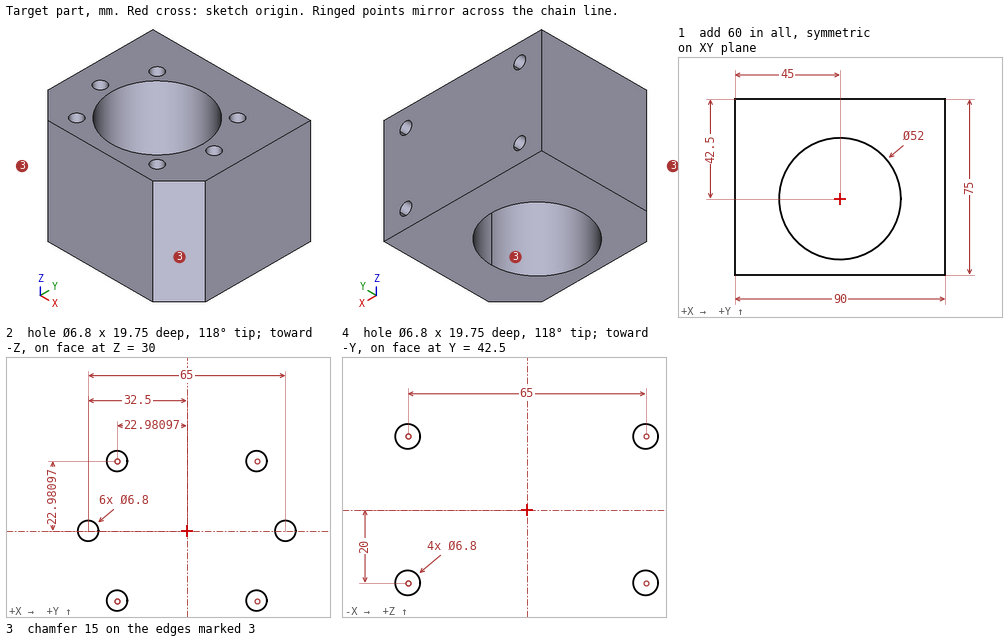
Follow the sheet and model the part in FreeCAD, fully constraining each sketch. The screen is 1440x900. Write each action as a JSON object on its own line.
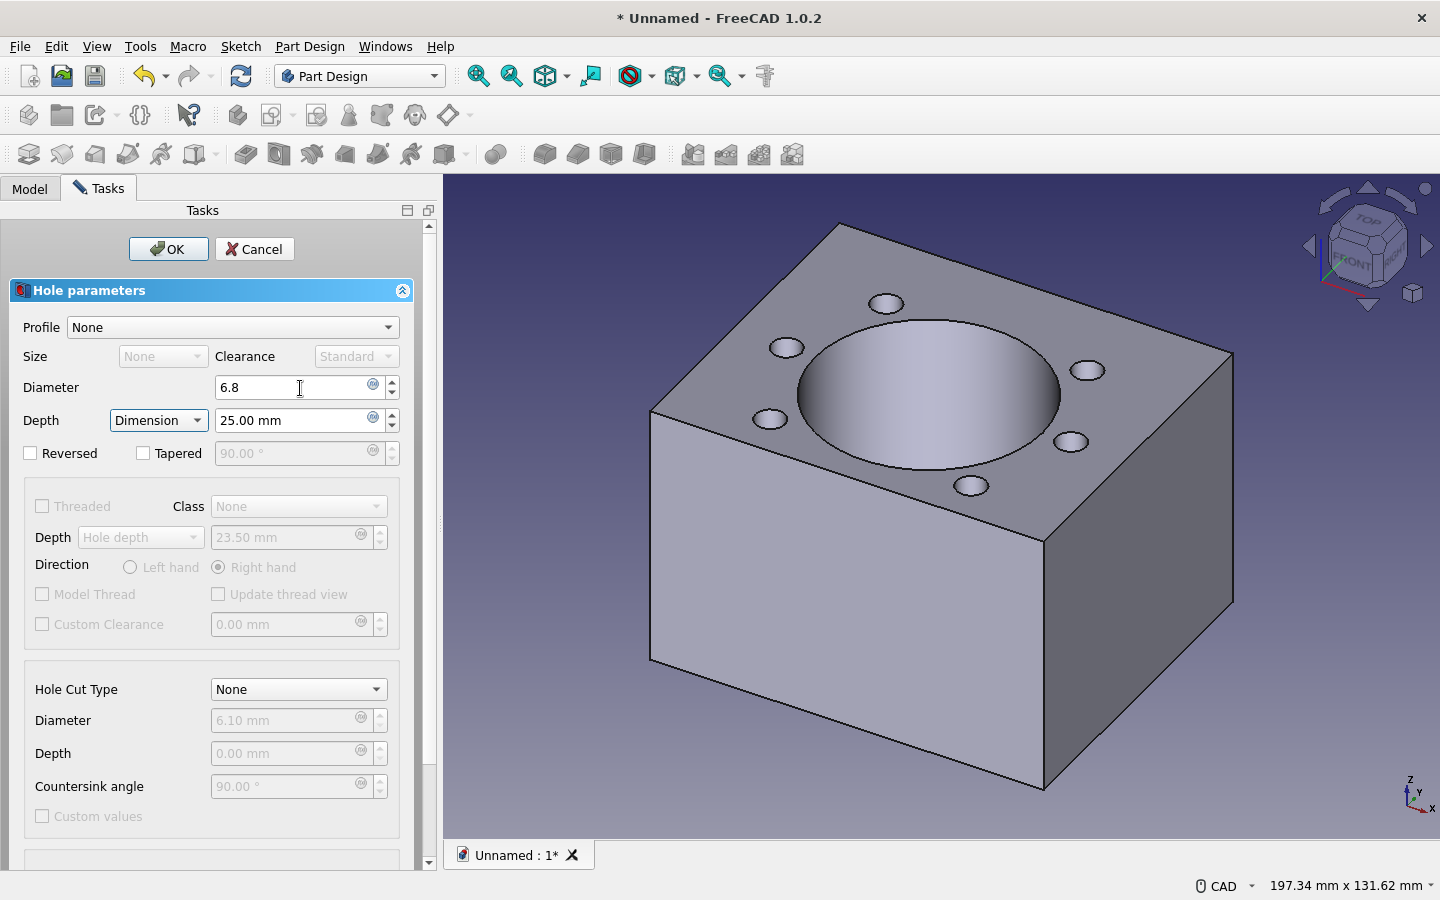
{"action": "triple_click", "coordinate": [300, 420]}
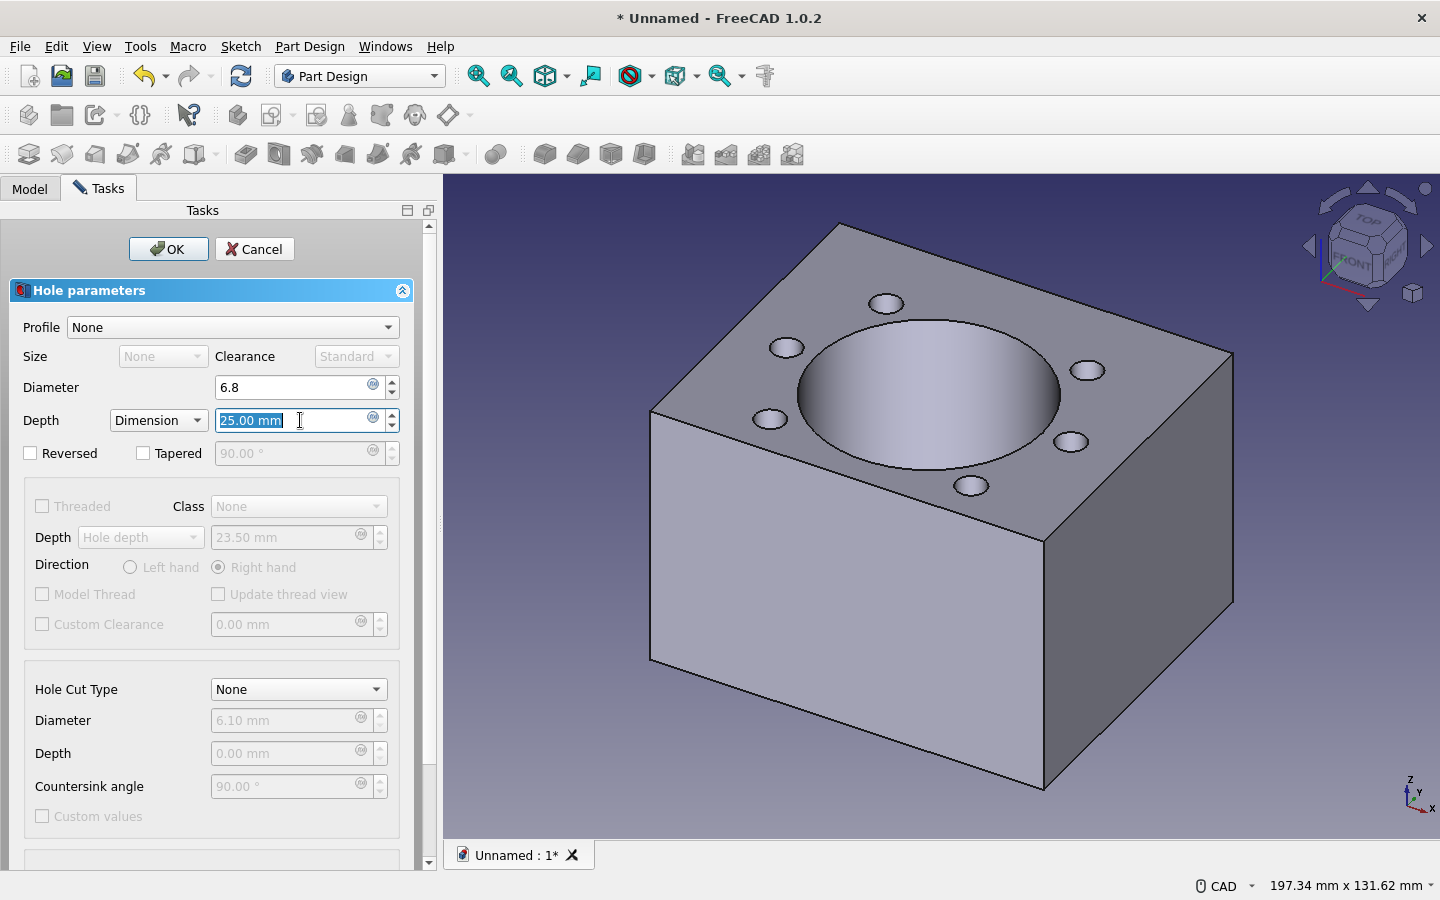
{"action": "type", "text": "19.75"}
{"action": "key", "text": "Tab"}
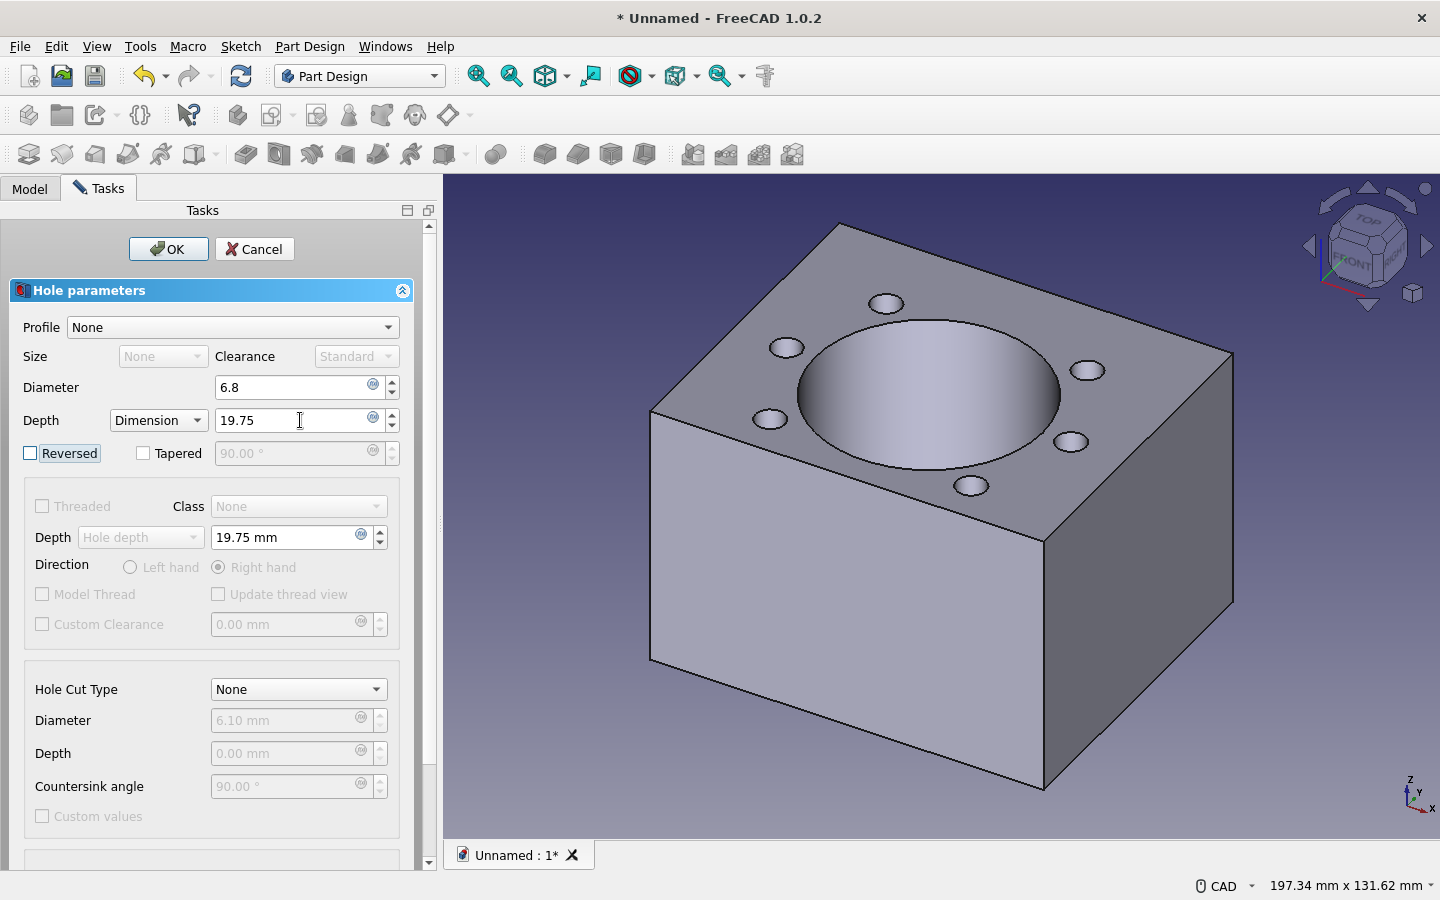
{"action": "left_click", "coordinate": [169, 249]}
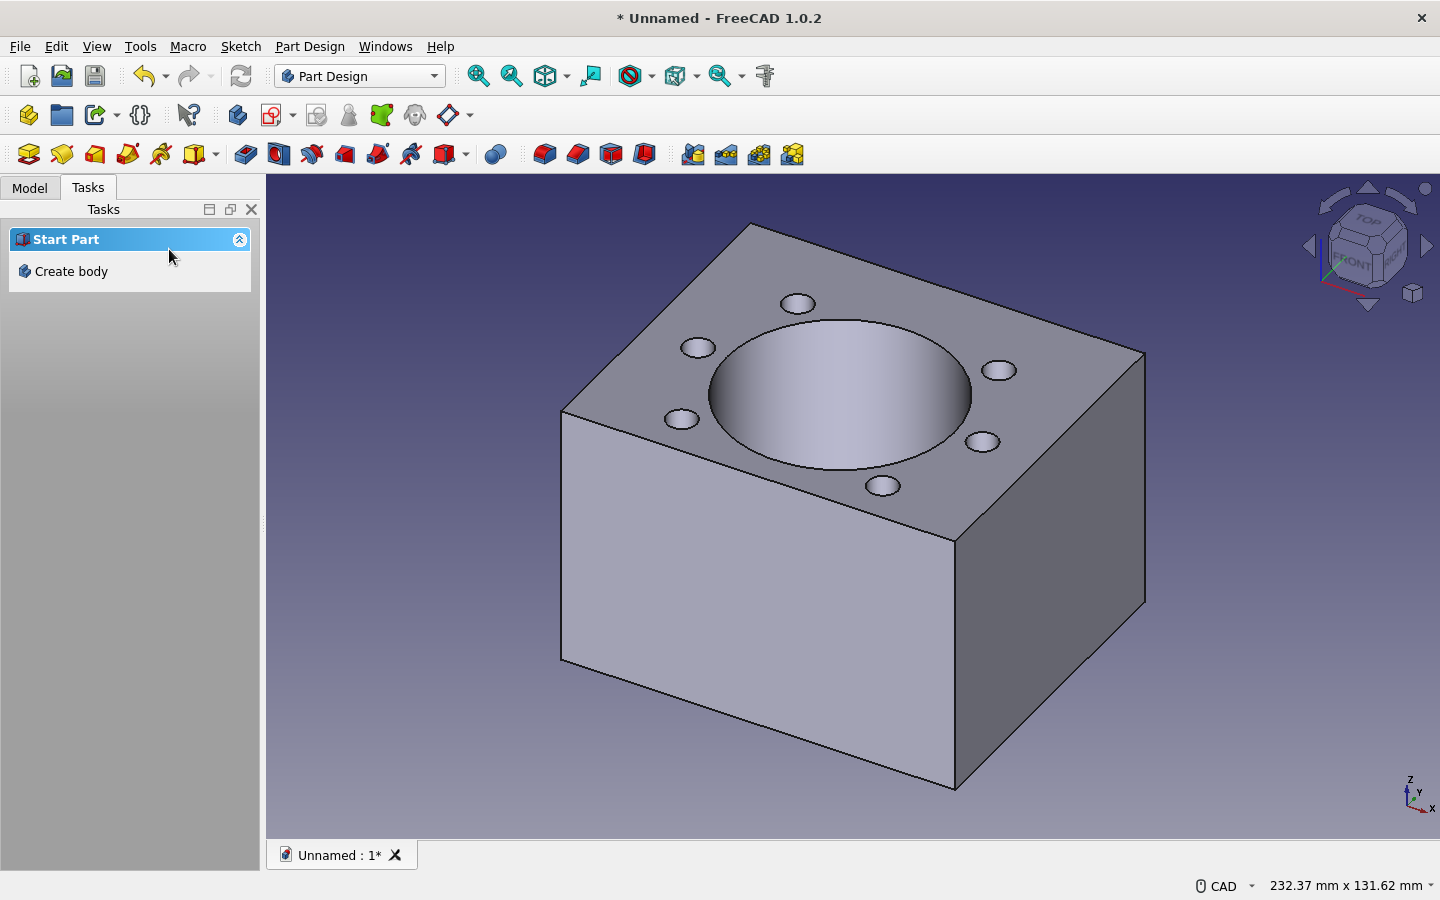
{"action": "left_click", "coordinate": [955, 665]}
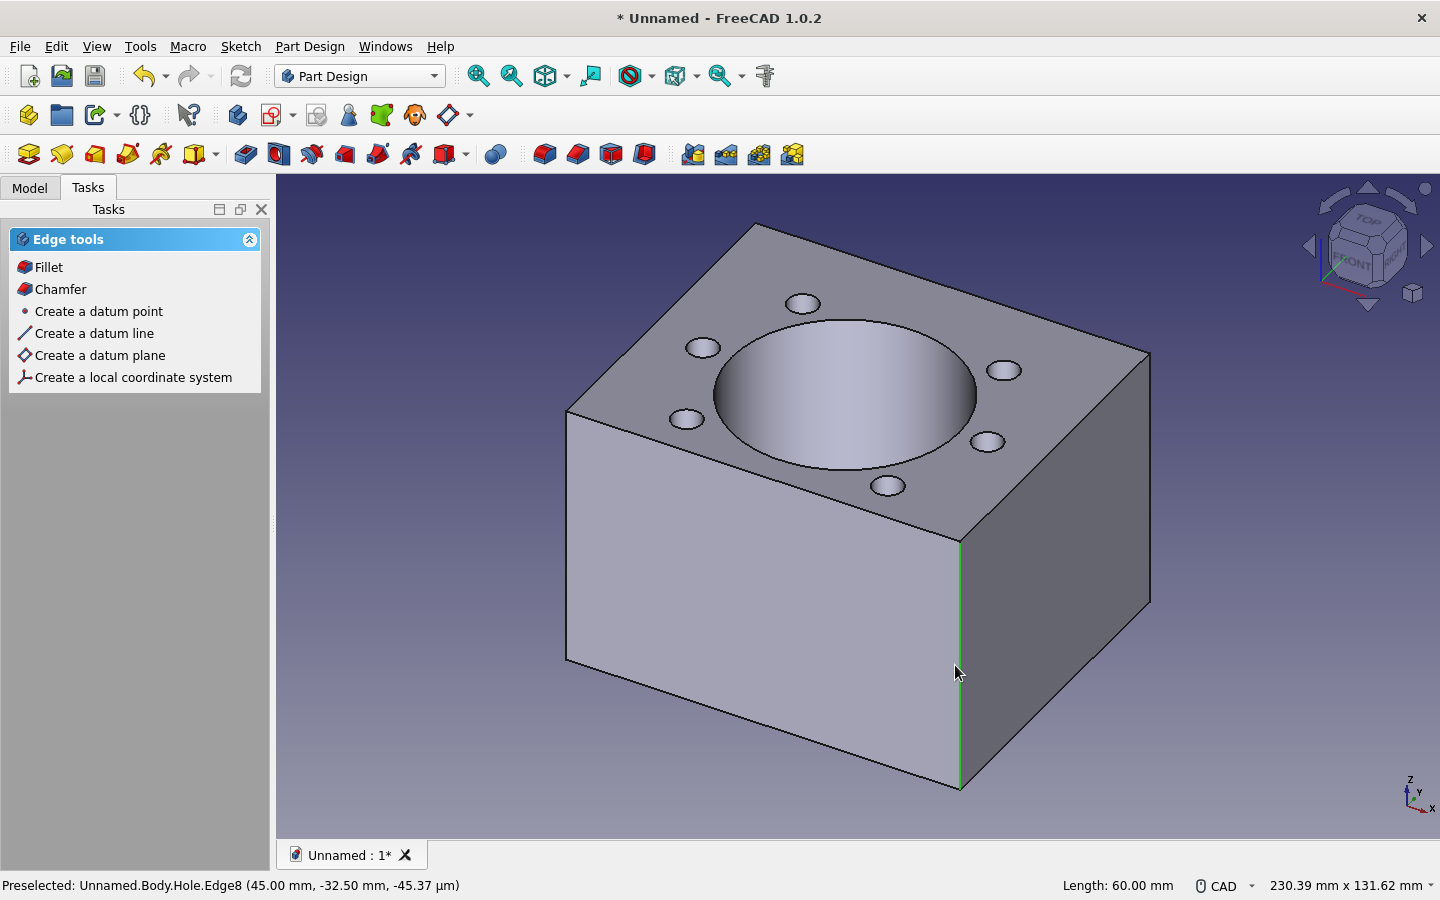
{"action": "key", "text": "0"}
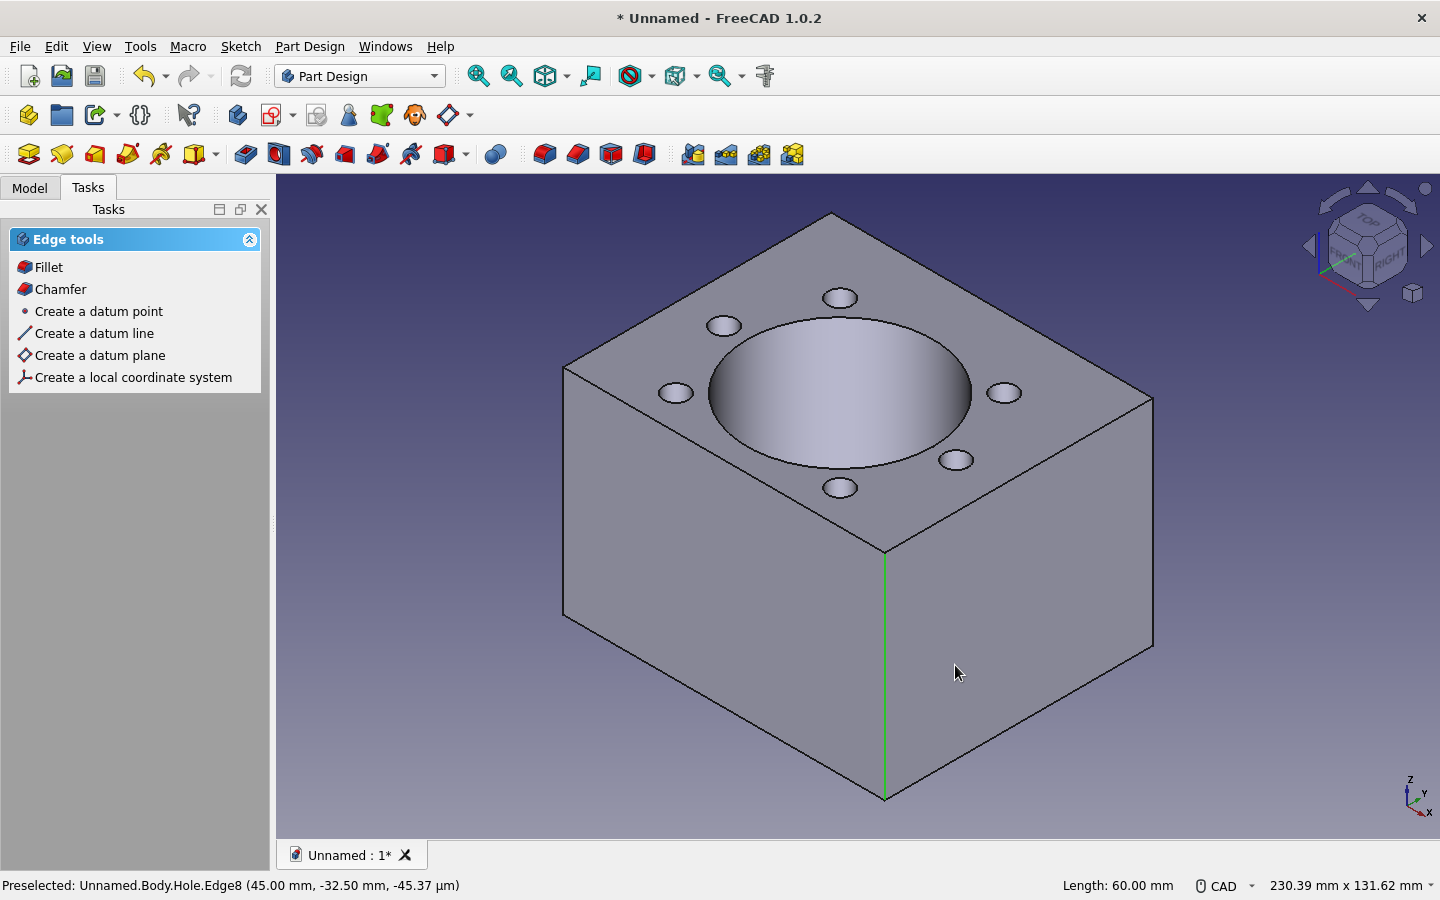
{"action": "key", "text": "2"}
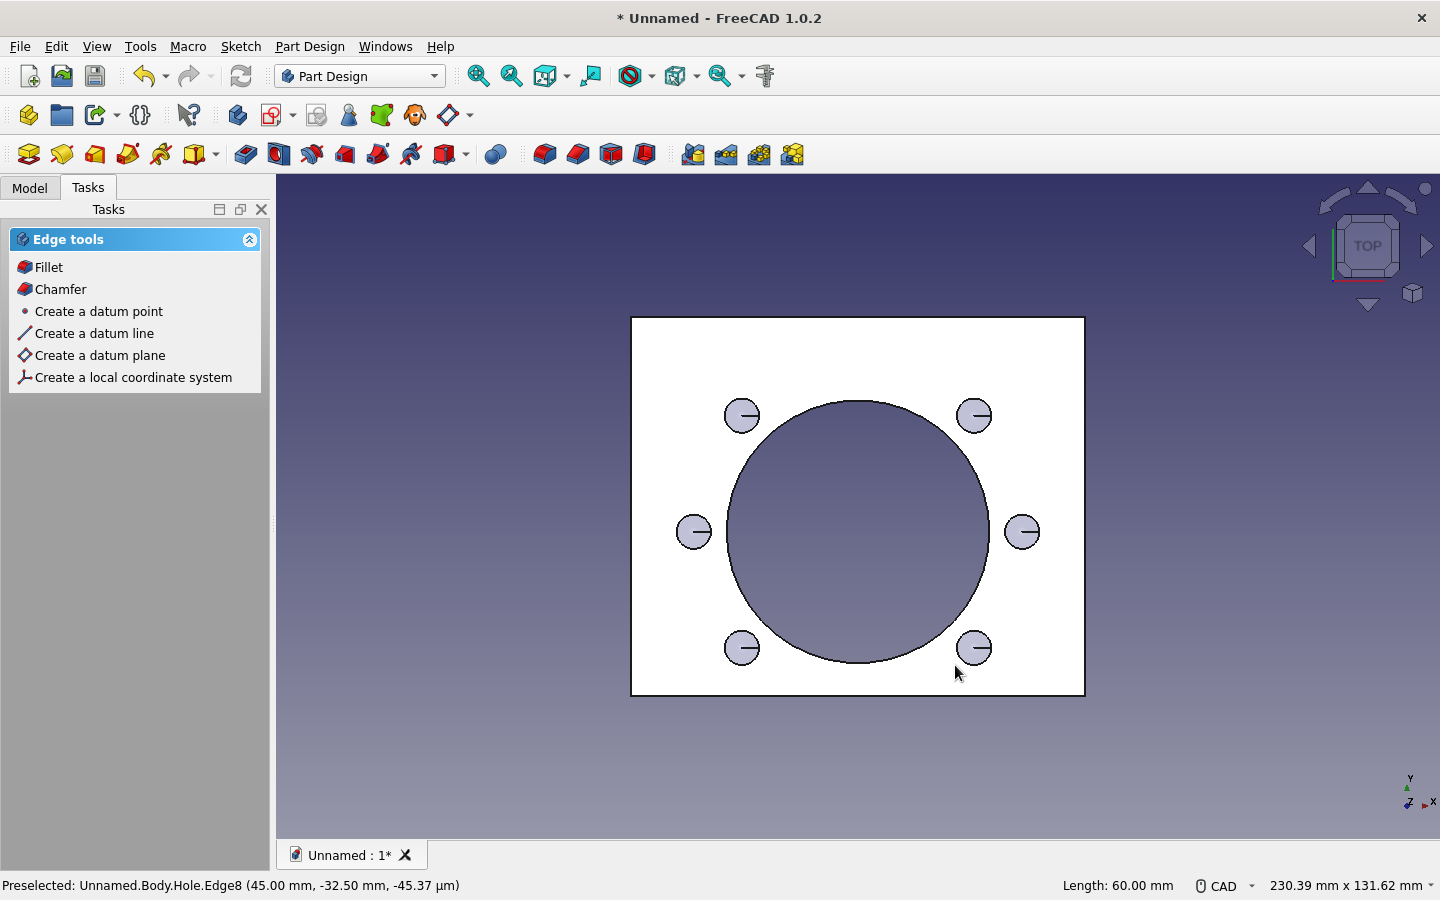
{"action": "key", "text": "1"}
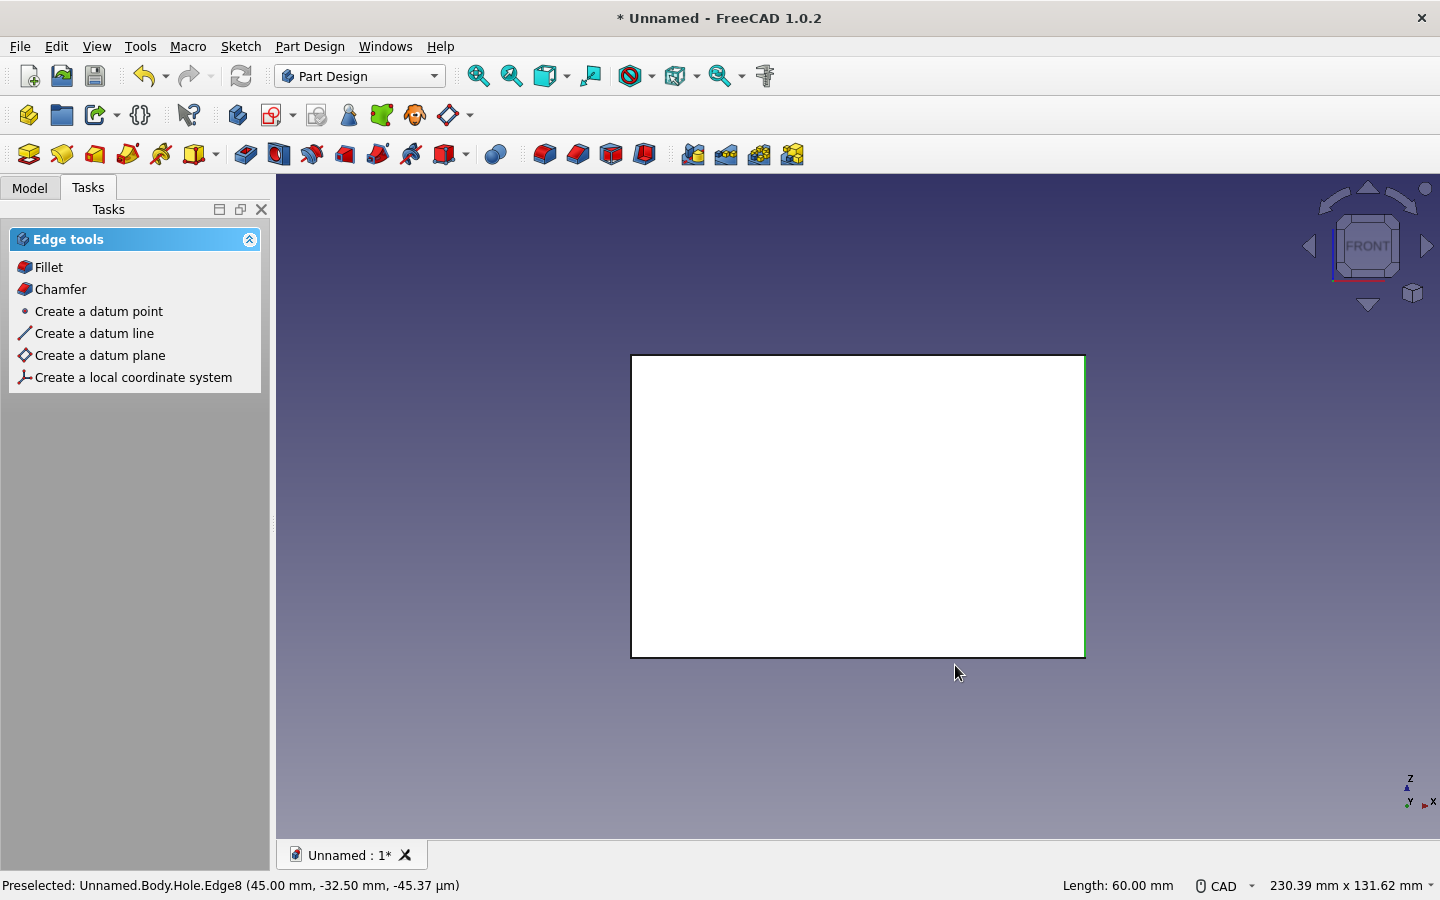
{"action": "left_click", "coordinate": [631, 506], "text": "ctrl"}